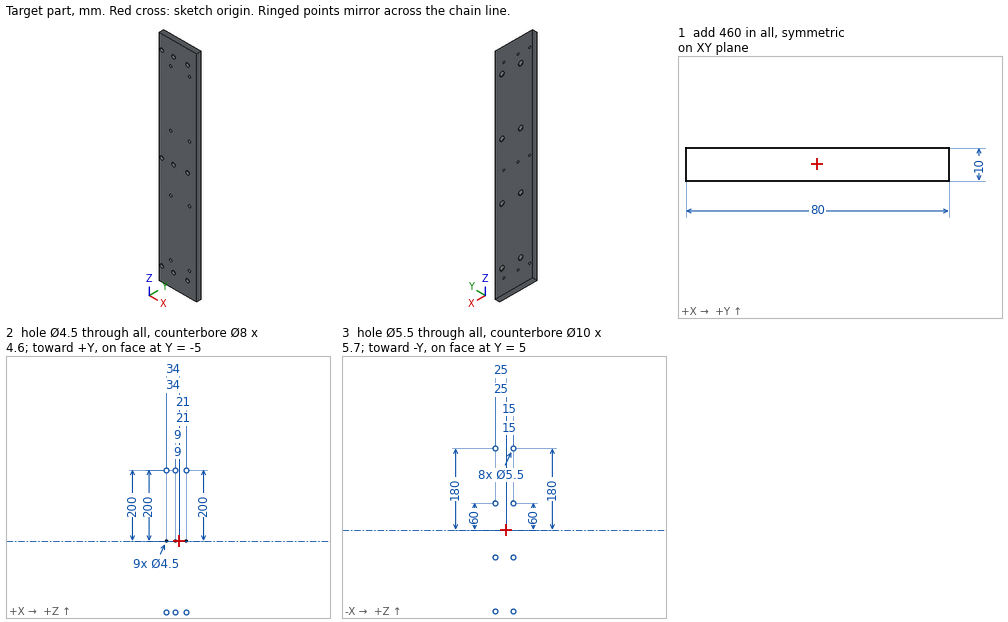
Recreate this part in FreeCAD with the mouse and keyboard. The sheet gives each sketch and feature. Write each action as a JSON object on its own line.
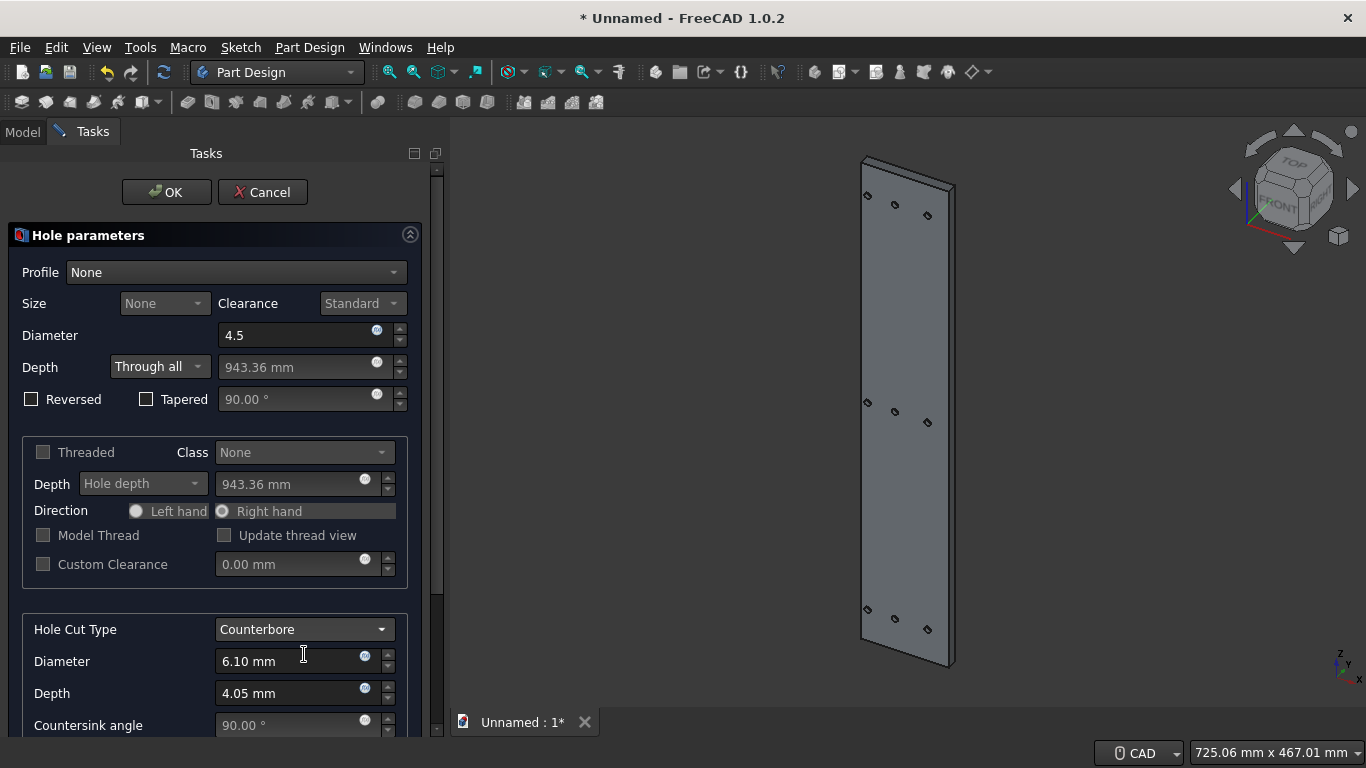
{"action": "triple_click", "coordinate": [298, 661]}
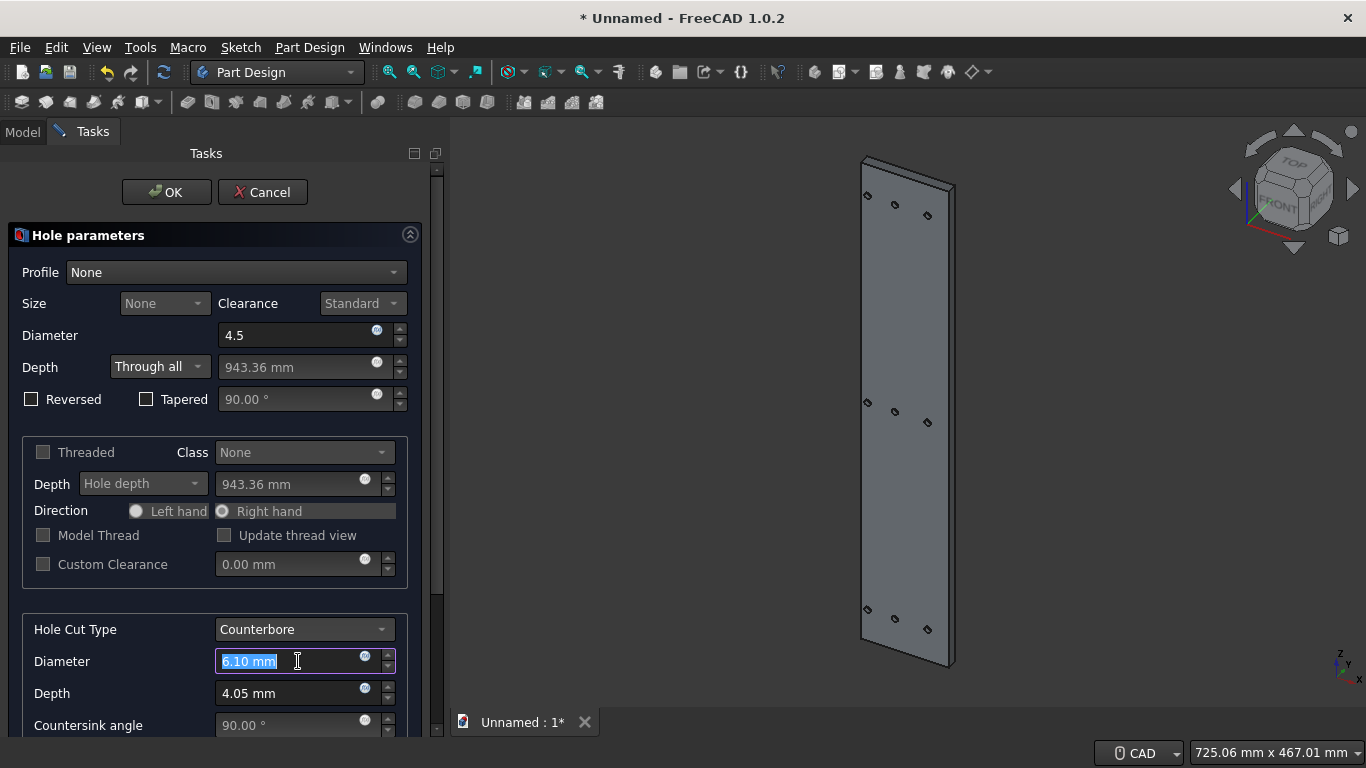
{"action": "type", "text": "8"}
{"action": "key", "text": "Tab"}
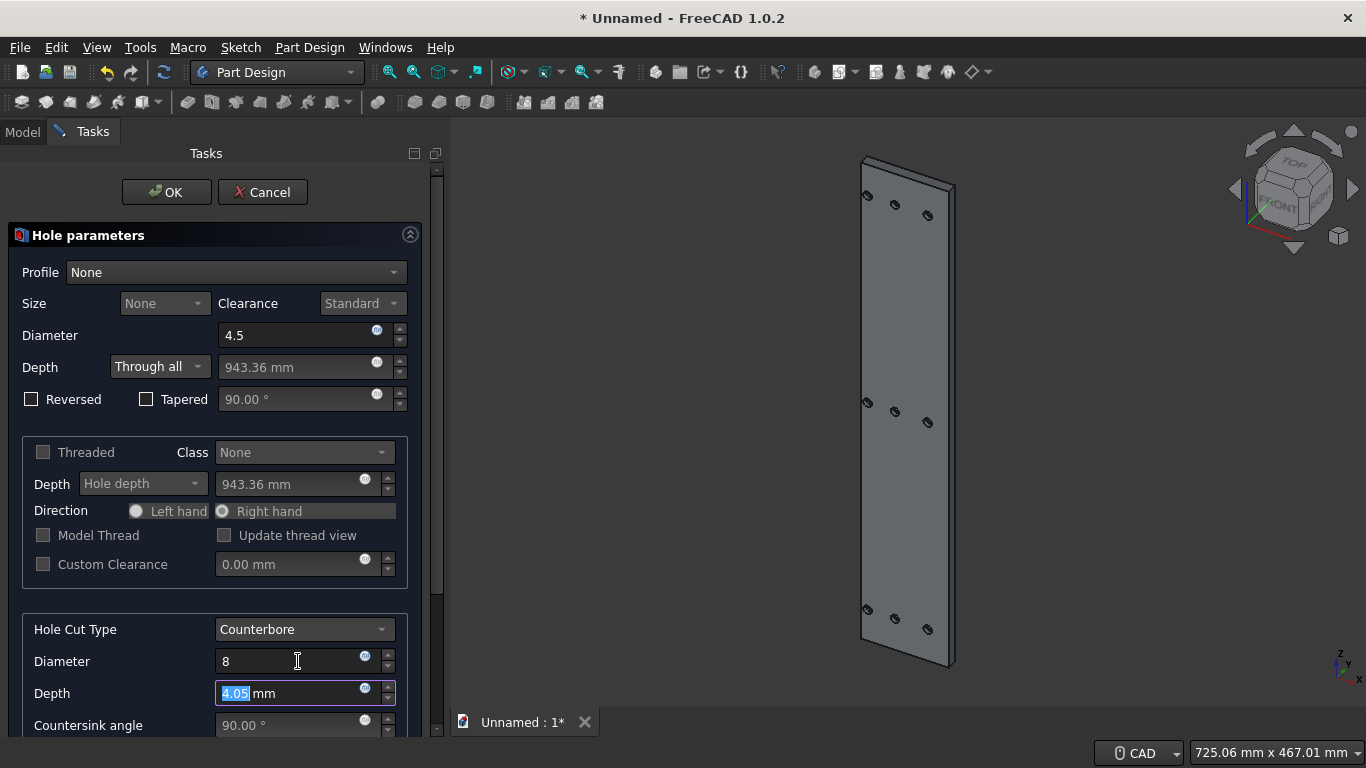
{"action": "type", "text": "4.6"}
{"action": "key", "text": "Tab"}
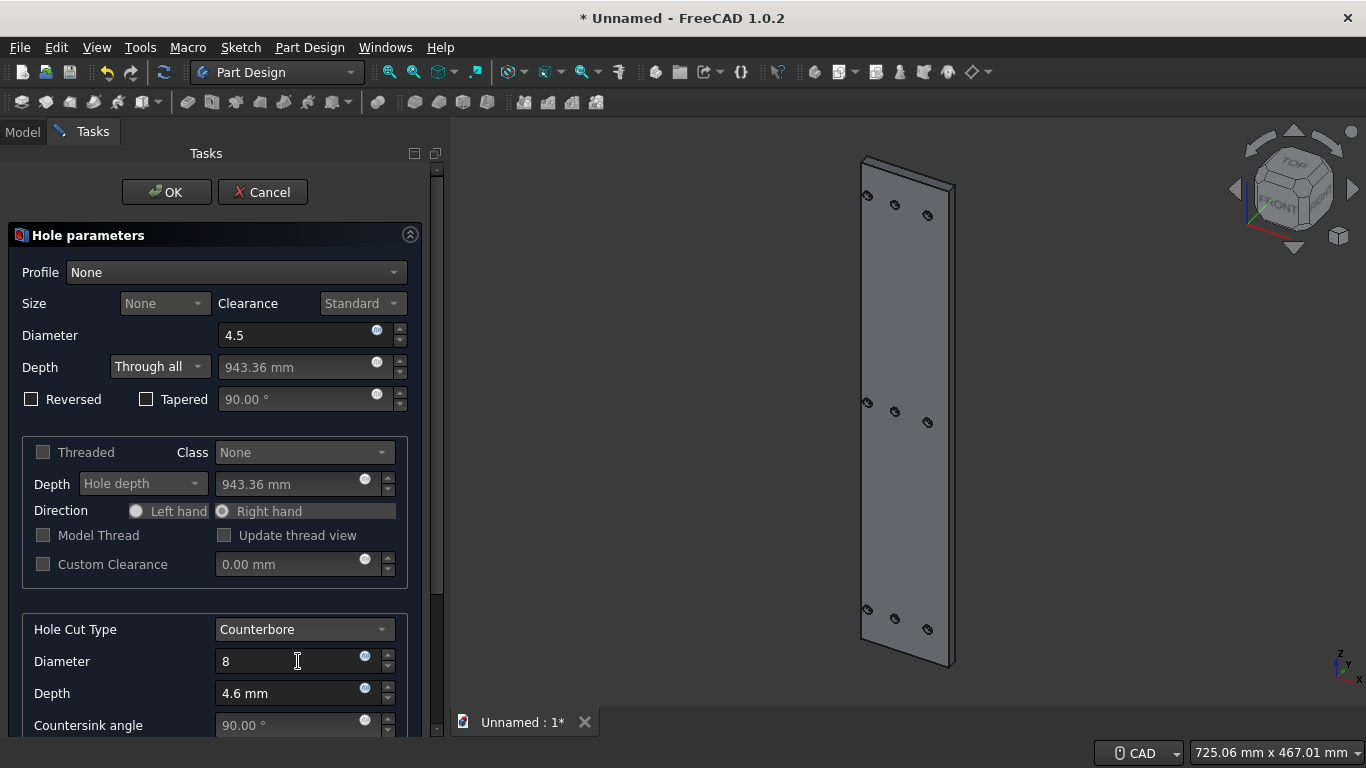
{"action": "left_click", "coordinate": [167, 192]}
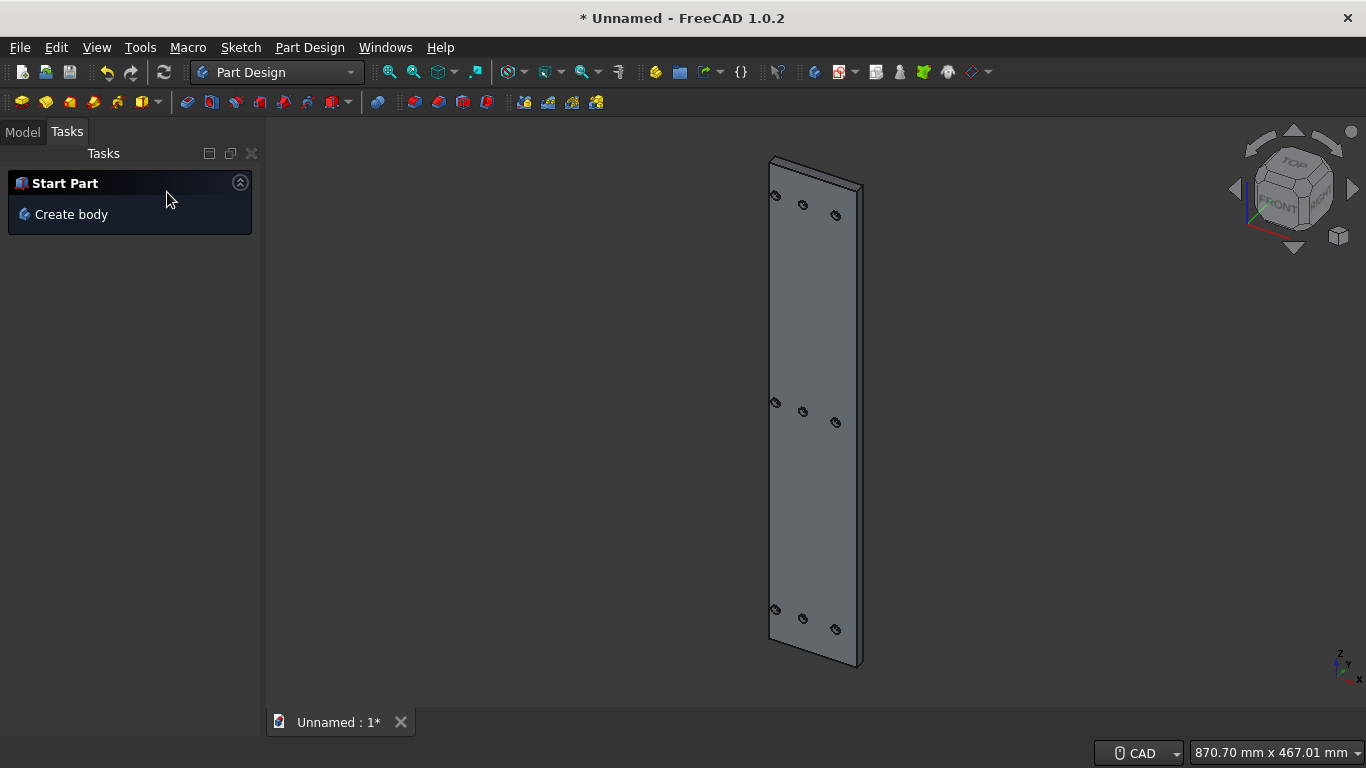
{"action": "key", "text": "4"}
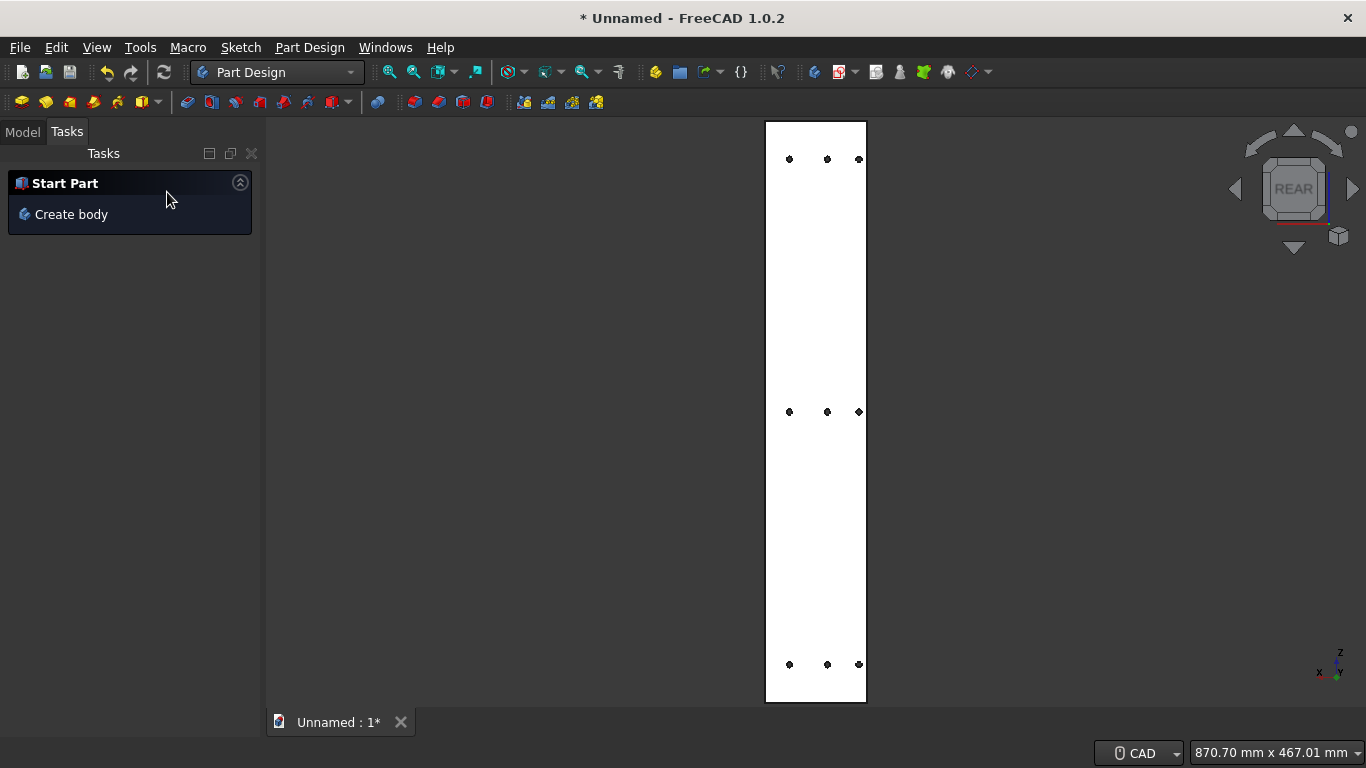
{"action": "left_click", "coordinate": [816, 245]}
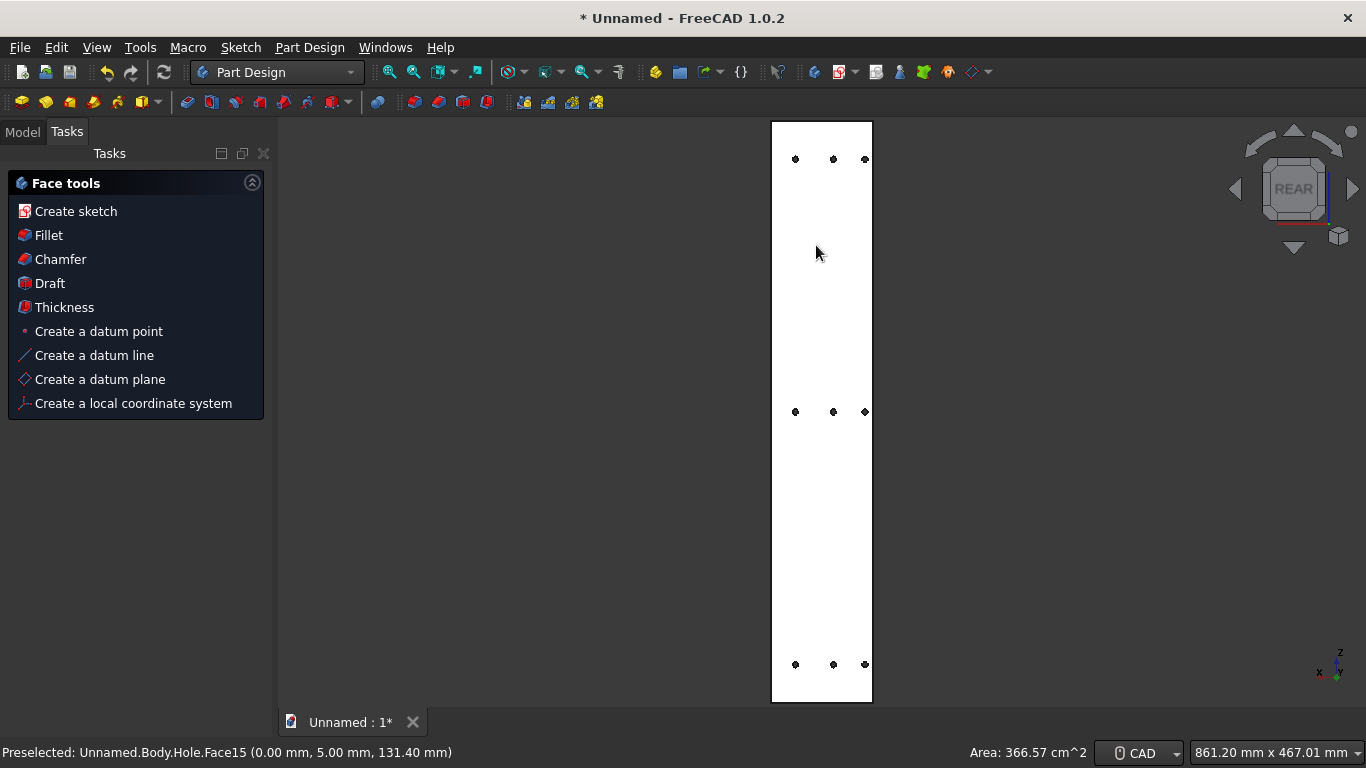
{"action": "left_click", "coordinate": [840, 72]}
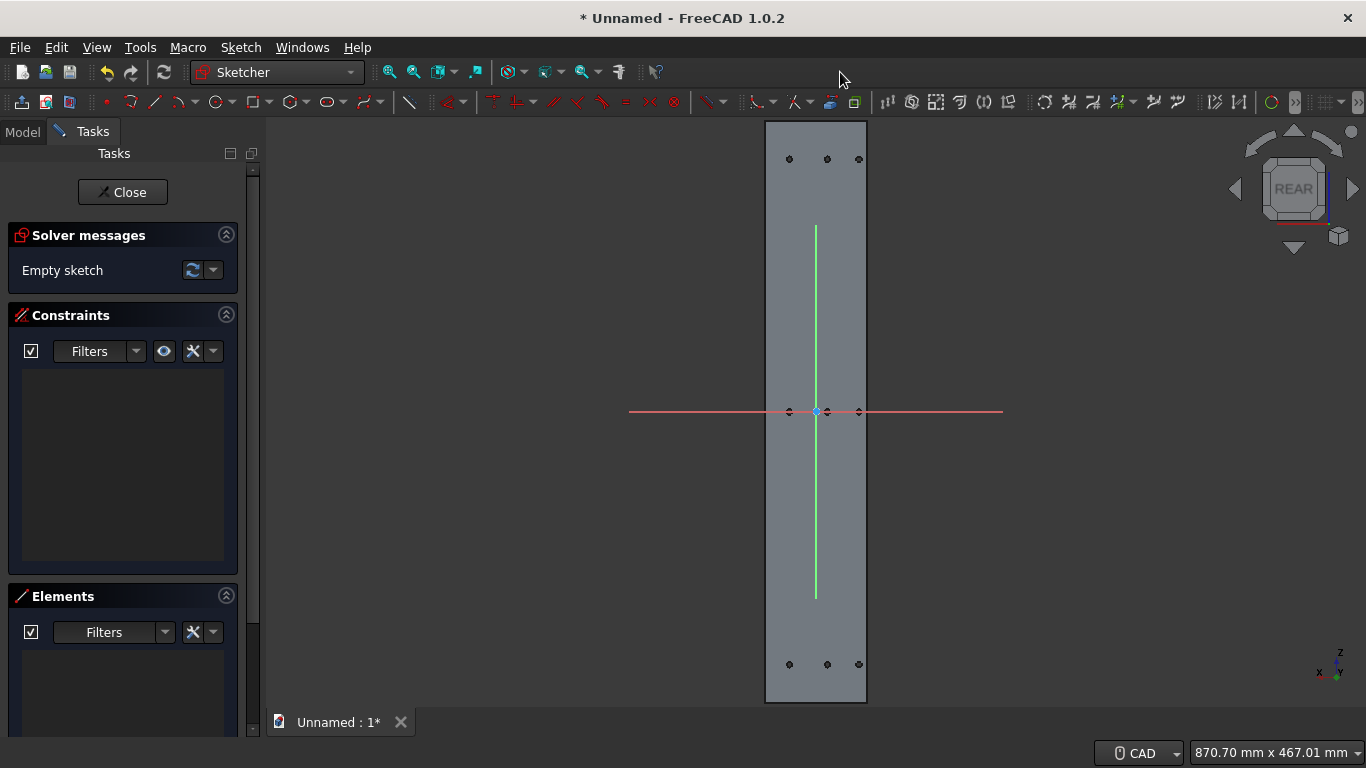
{"action": "left_click", "coordinate": [216, 102]}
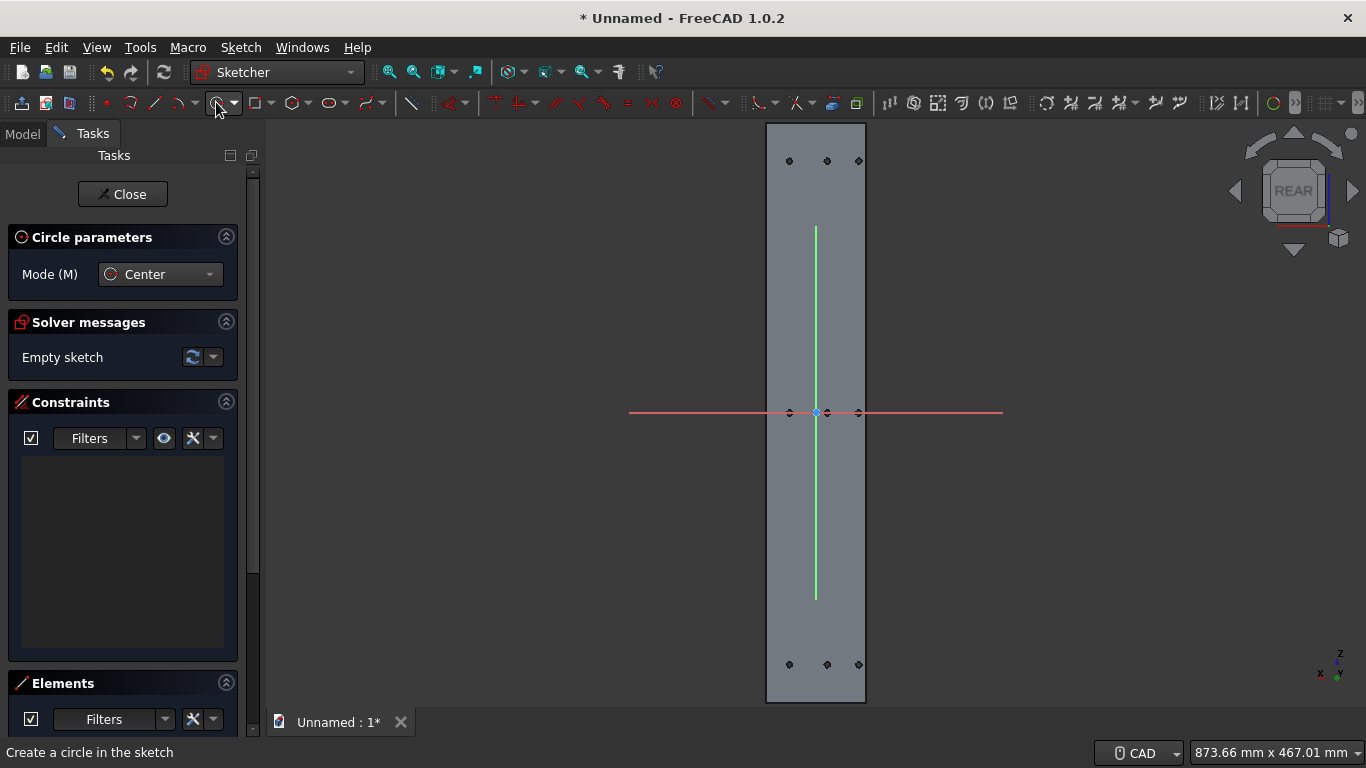
{"action": "scroll", "coordinate": [835, 186], "scroll_direction": "up", "scroll_amount": 10}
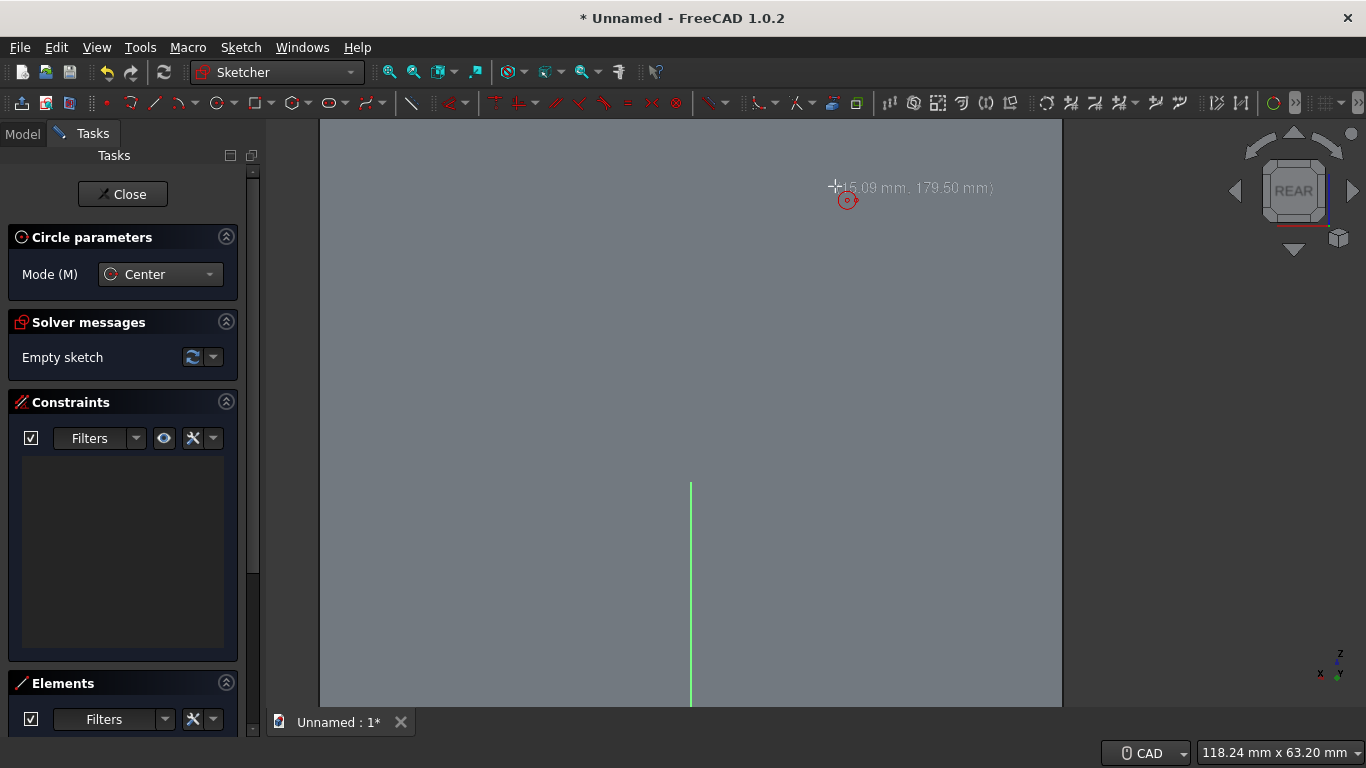
{"action": "scroll", "coordinate": [760, 232], "scroll_direction": "down", "scroll_amount": 11}